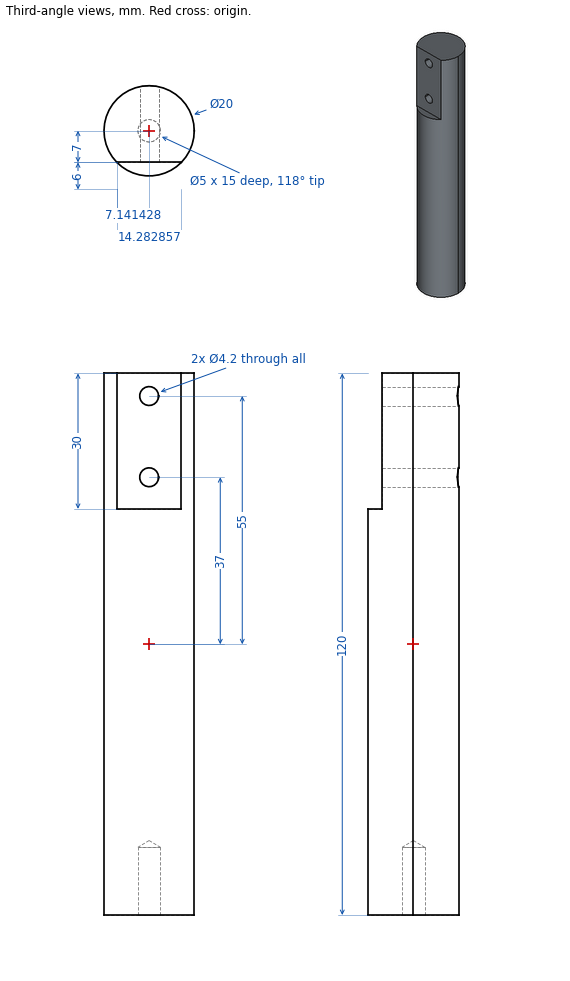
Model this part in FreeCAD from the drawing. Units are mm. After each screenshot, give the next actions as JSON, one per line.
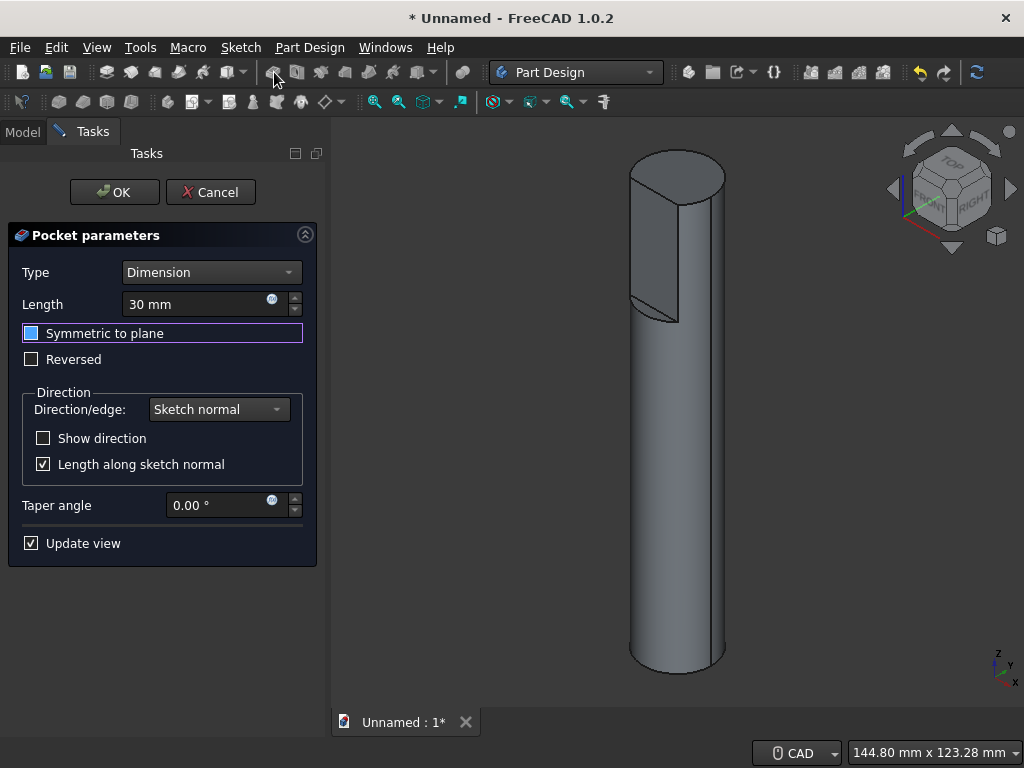
{"action": "left_click", "coordinate": [115, 192]}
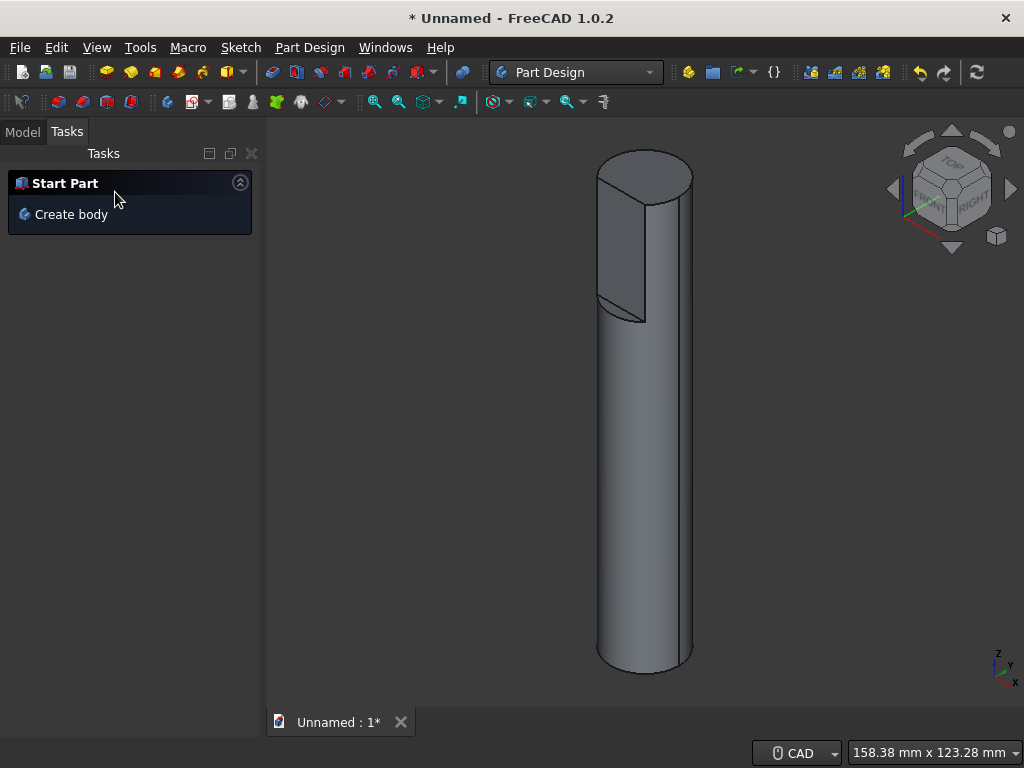
{"action": "left_click", "coordinate": [621, 232]}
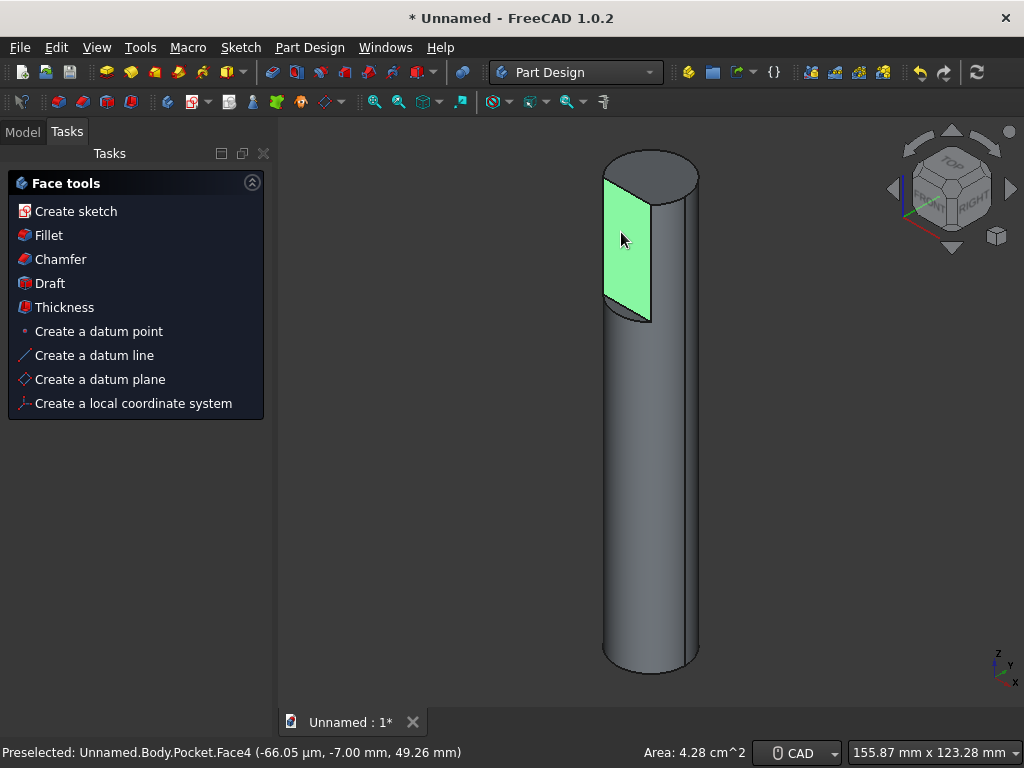
{"action": "left_click", "coordinate": [192, 102]}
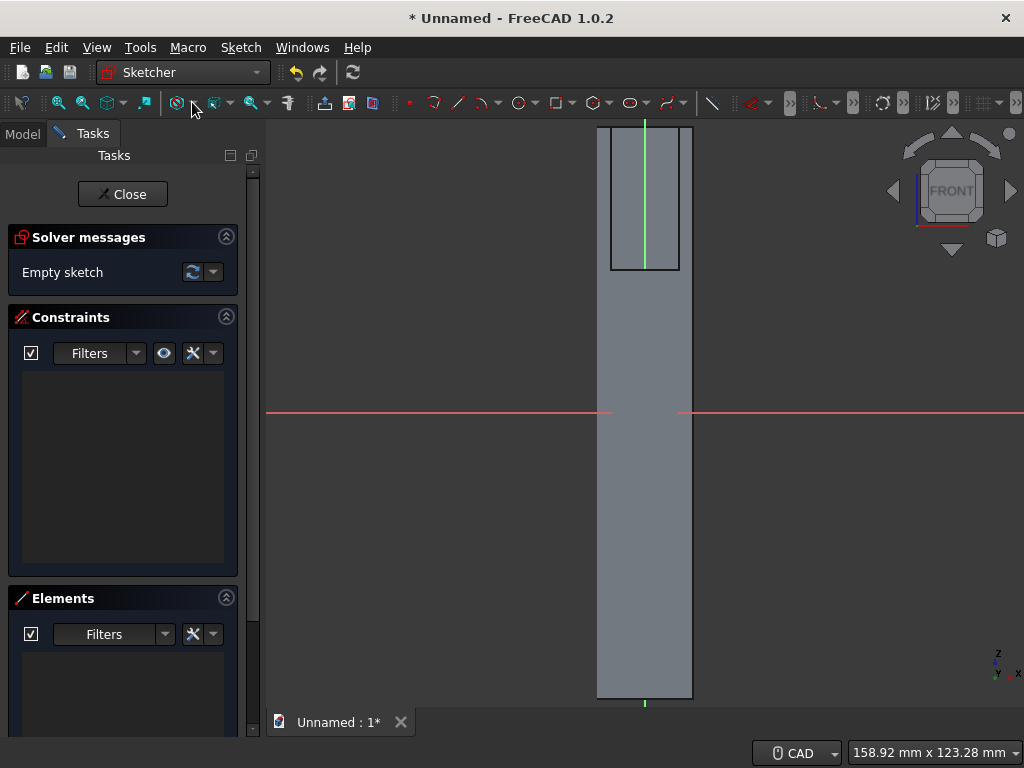
{"action": "scroll", "coordinate": [576, 413], "scroll_direction": "down", "scroll_amount": 5}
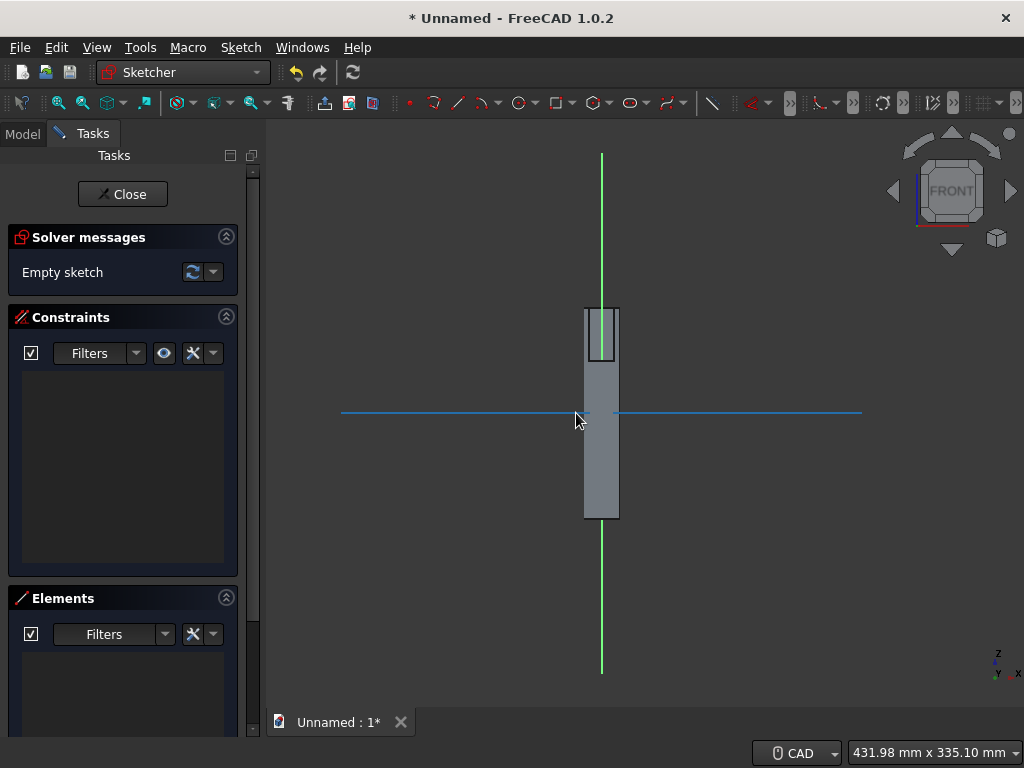
{"action": "scroll", "coordinate": [605, 323], "scroll_direction": "up", "scroll_amount": 11}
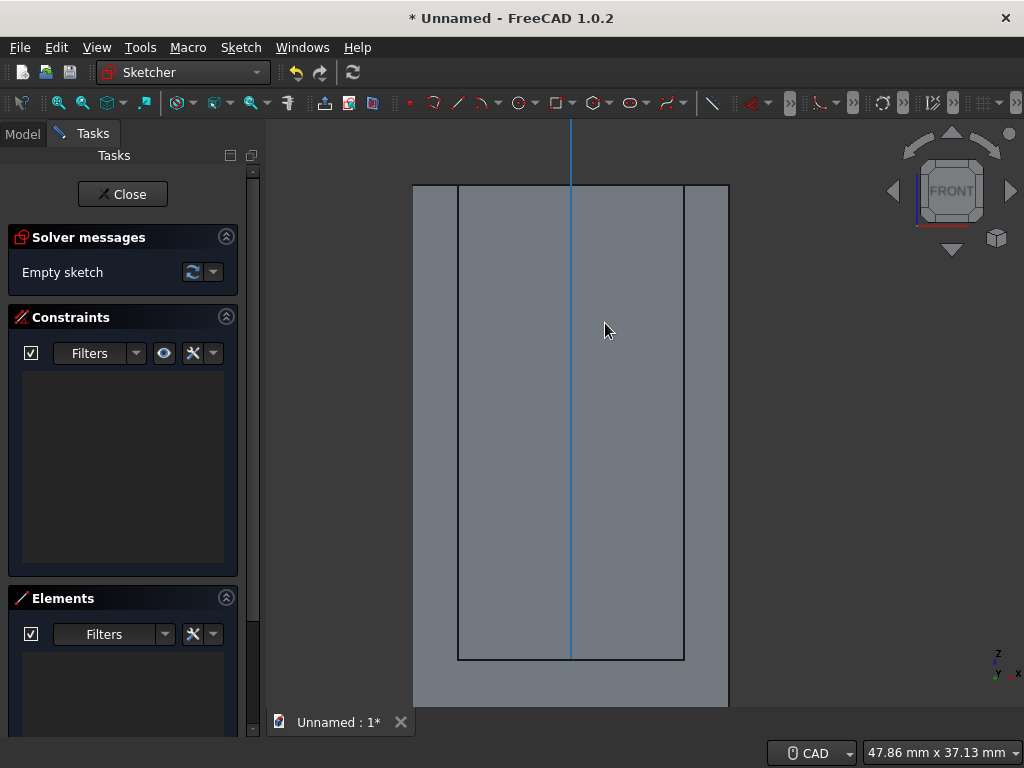
{"action": "left_click", "coordinate": [520, 104]}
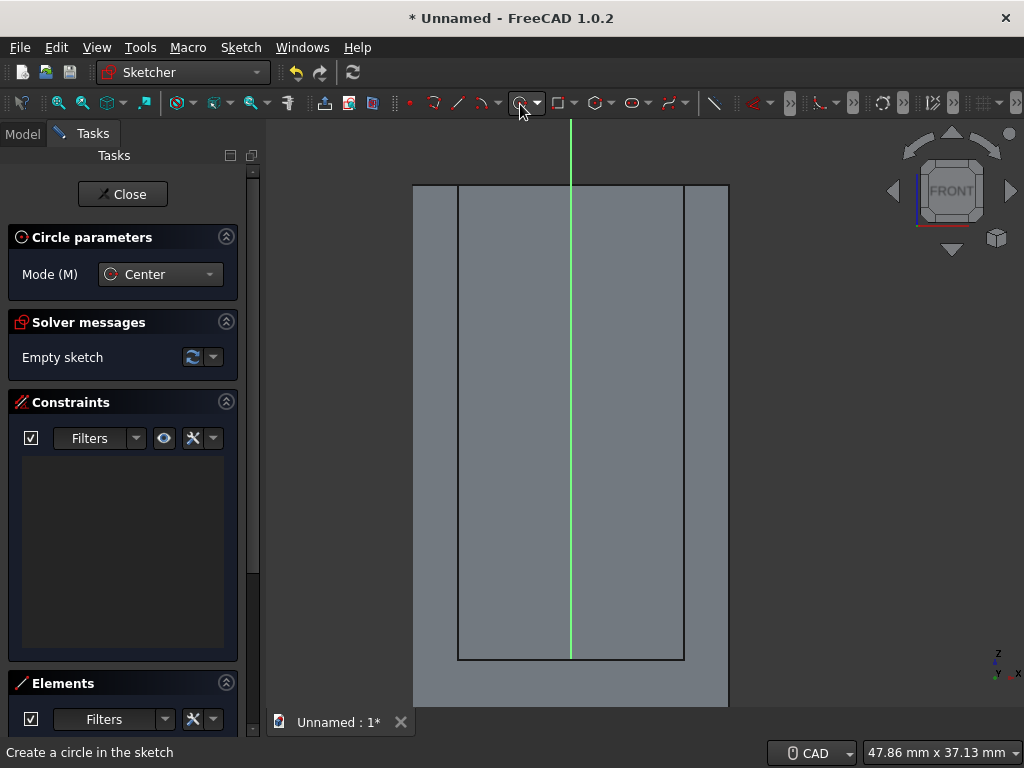
{"action": "left_click", "coordinate": [571, 264]}
{"action": "left_click", "coordinate": [594, 241]}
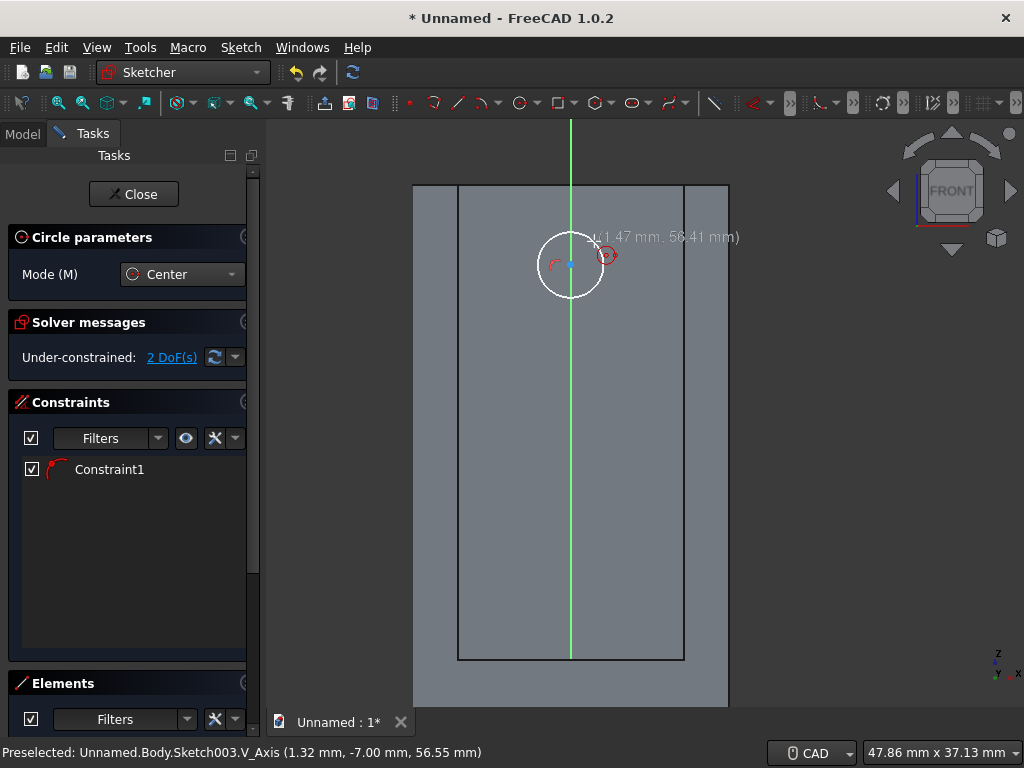
{"action": "left_click", "coordinate": [571, 549]}
{"action": "left_click", "coordinate": [594, 526]}
{"action": "key", "text": "Escape"}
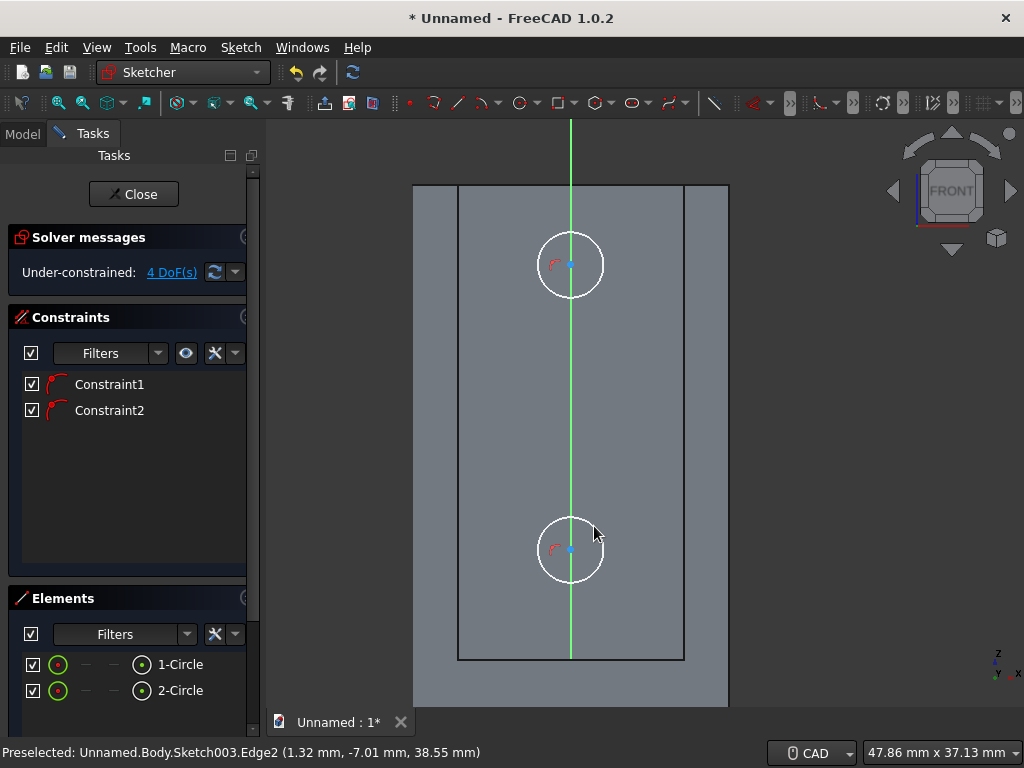
{"action": "left_click", "coordinate": [594, 242]}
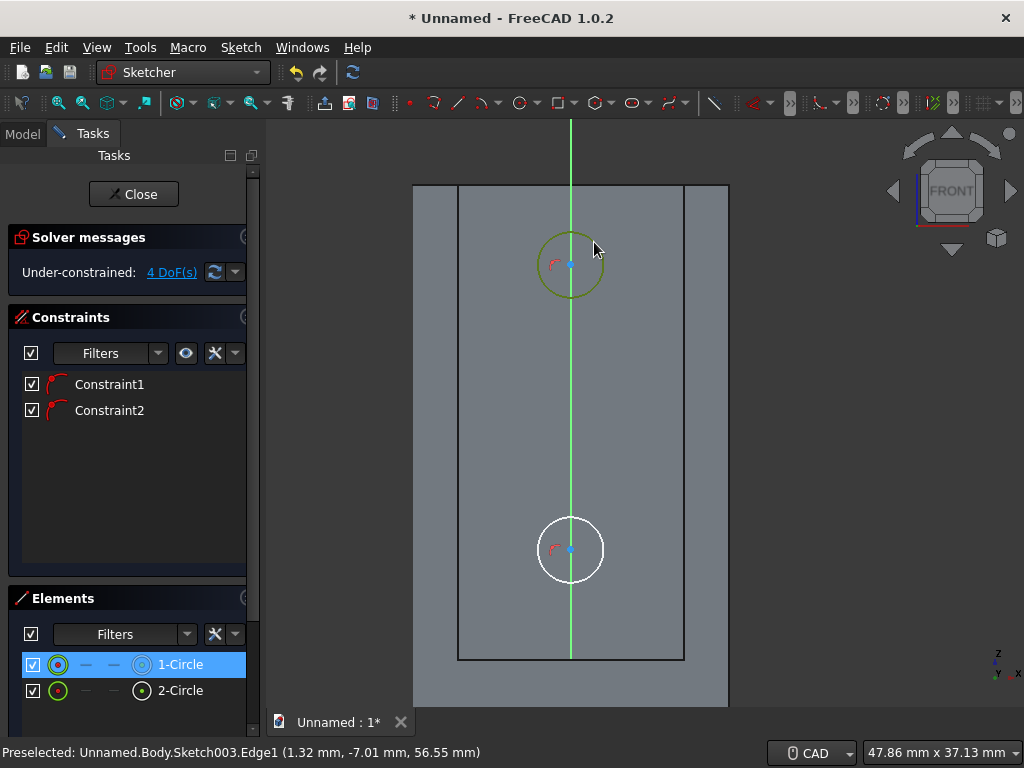
{"action": "left_click", "coordinate": [594, 527]}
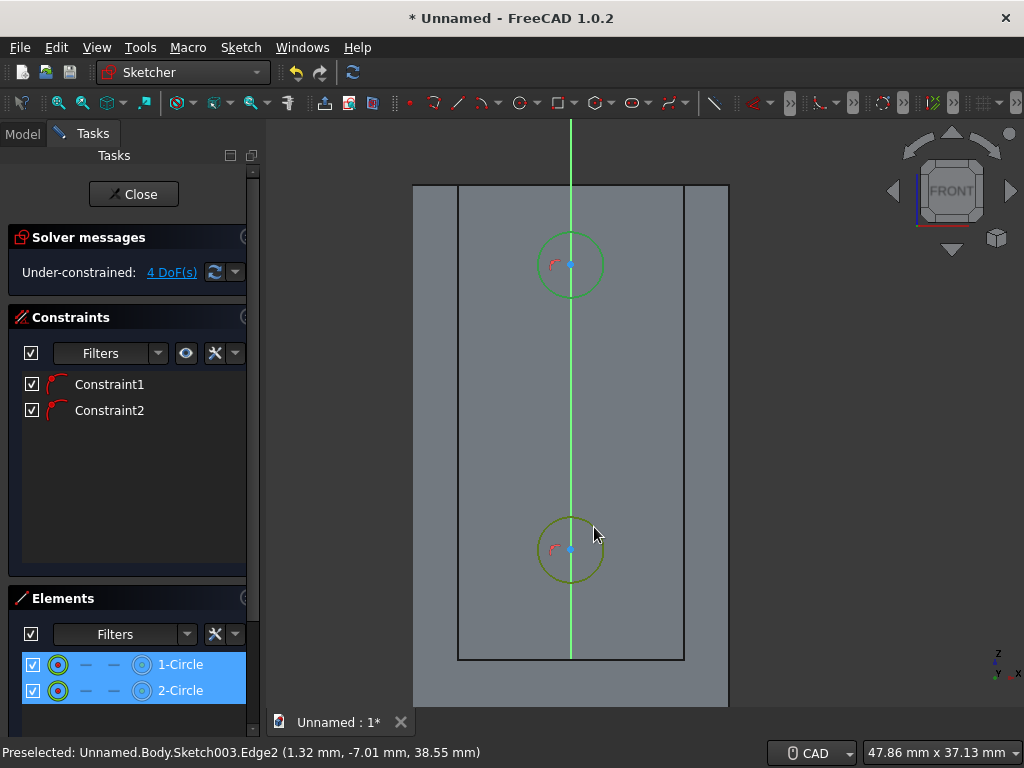
{"action": "key", "text": "e"}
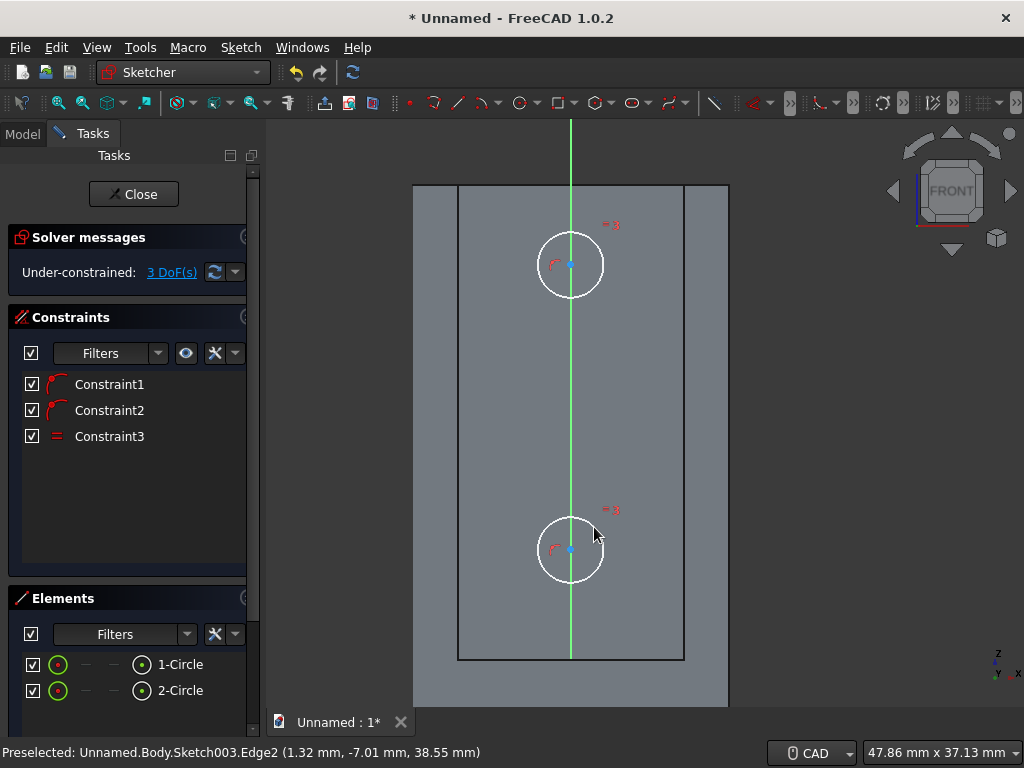
{"action": "left_click", "coordinate": [754, 104]}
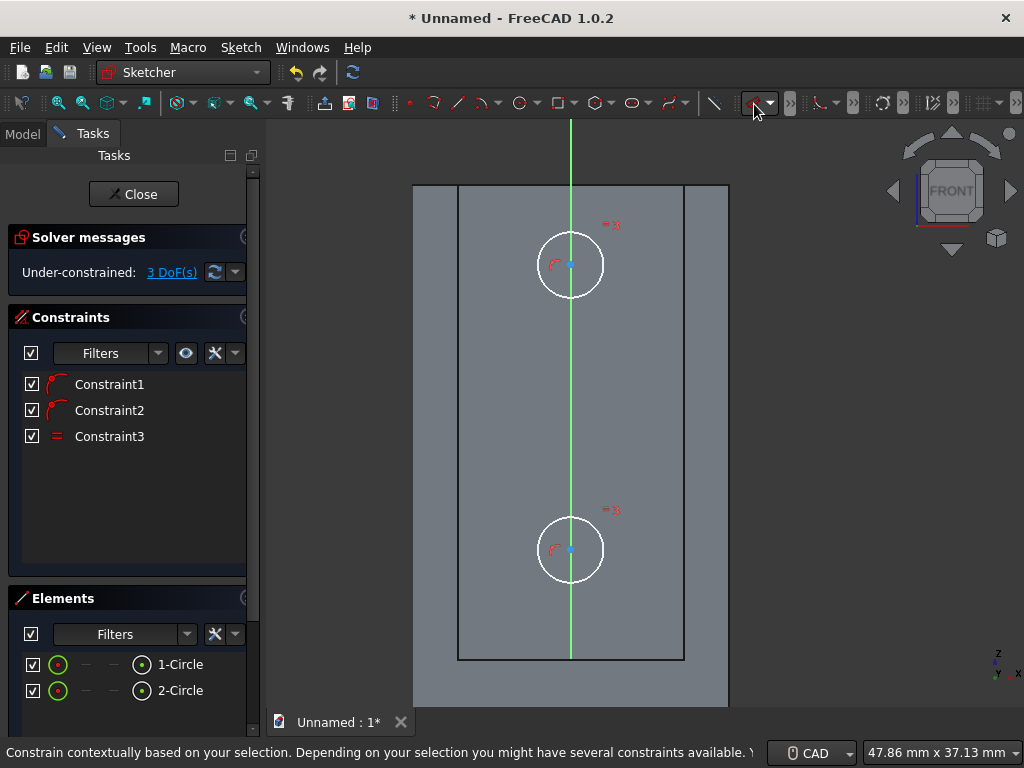
{"action": "left_click", "coordinate": [594, 242]}
{"action": "left_click", "coordinate": [617, 220]}